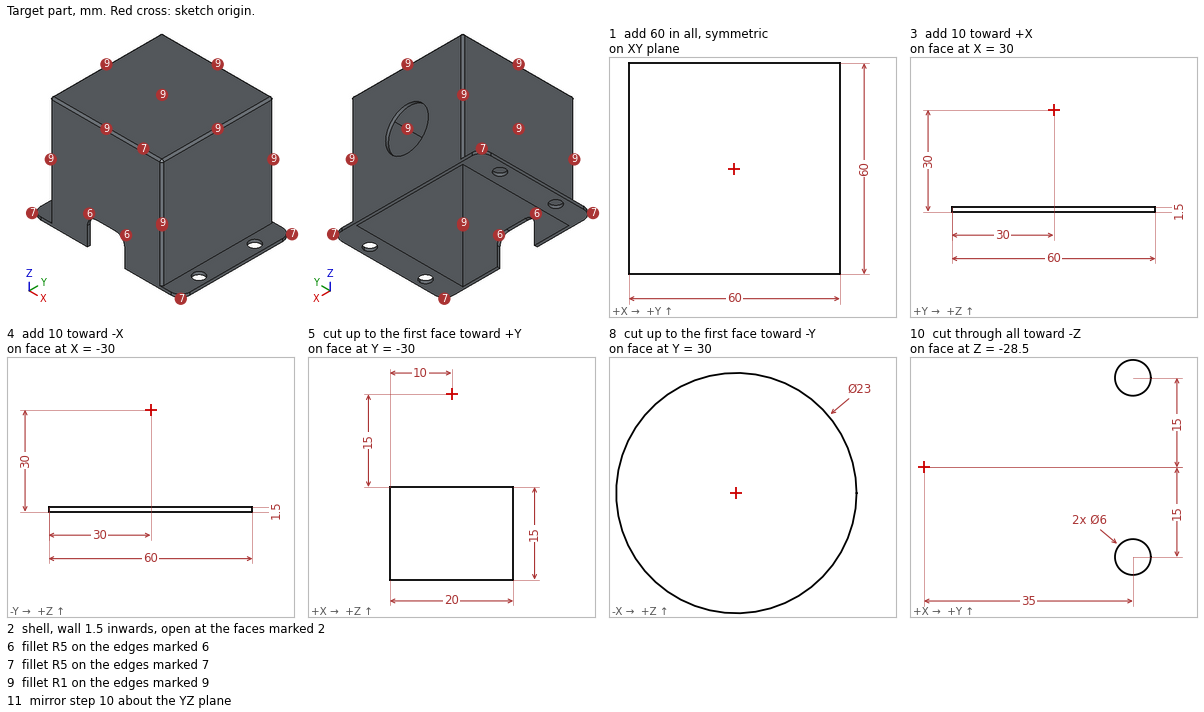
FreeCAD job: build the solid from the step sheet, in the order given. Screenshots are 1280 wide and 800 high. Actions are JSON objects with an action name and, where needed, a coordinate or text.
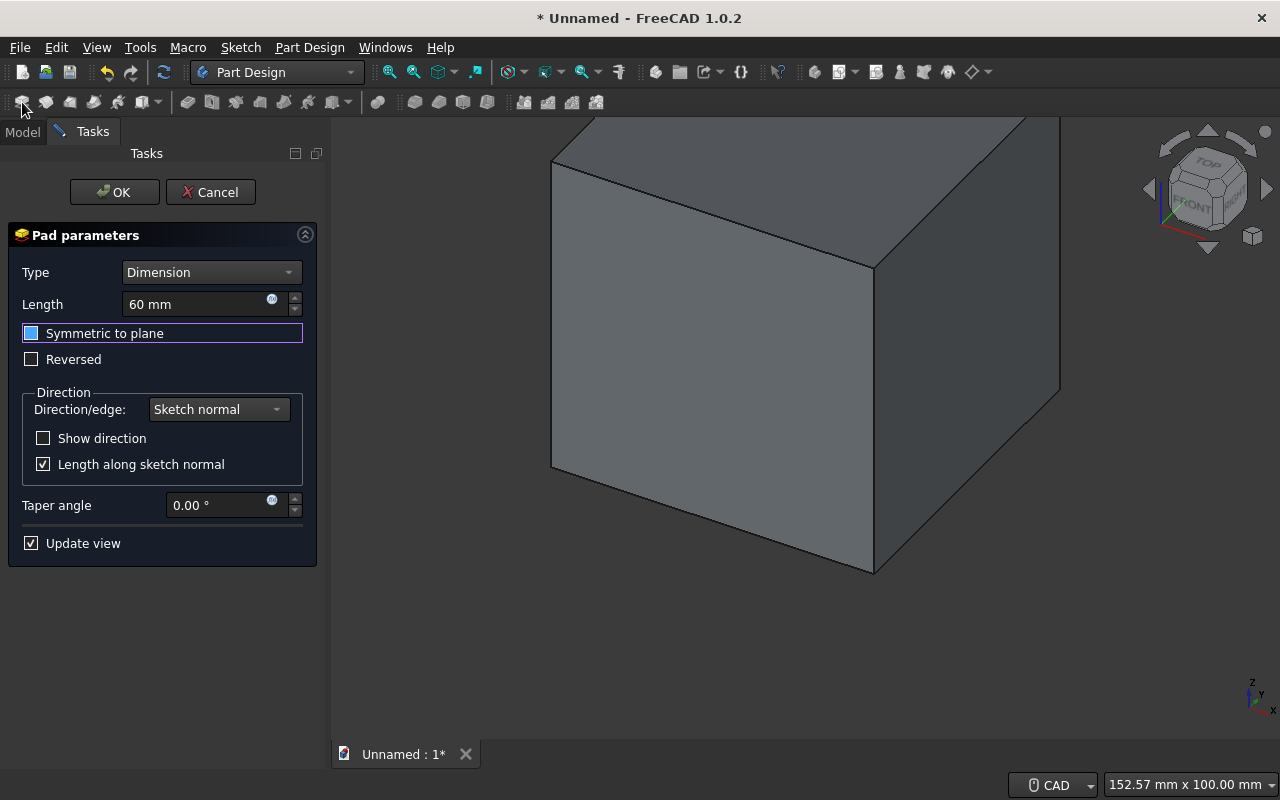
{"action": "left_click", "coordinate": [30, 333]}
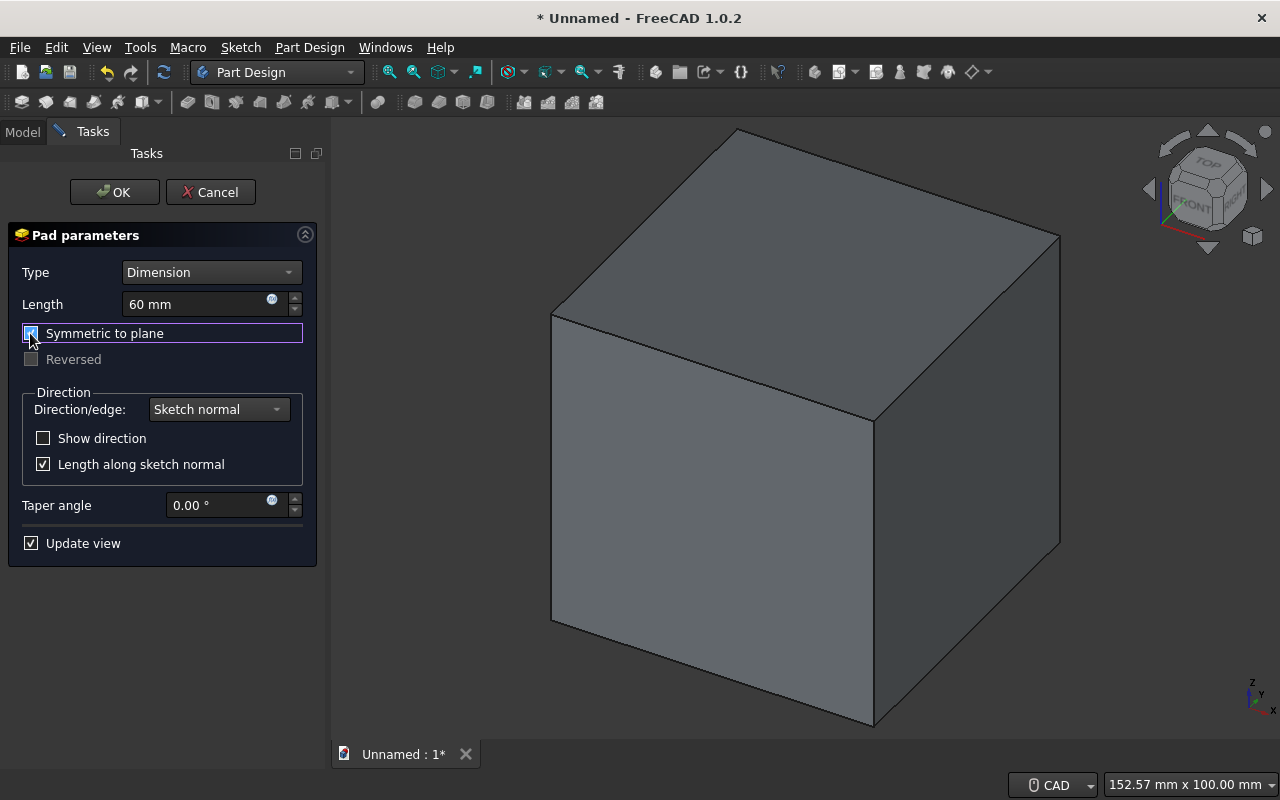
{"action": "left_click", "coordinate": [115, 192]}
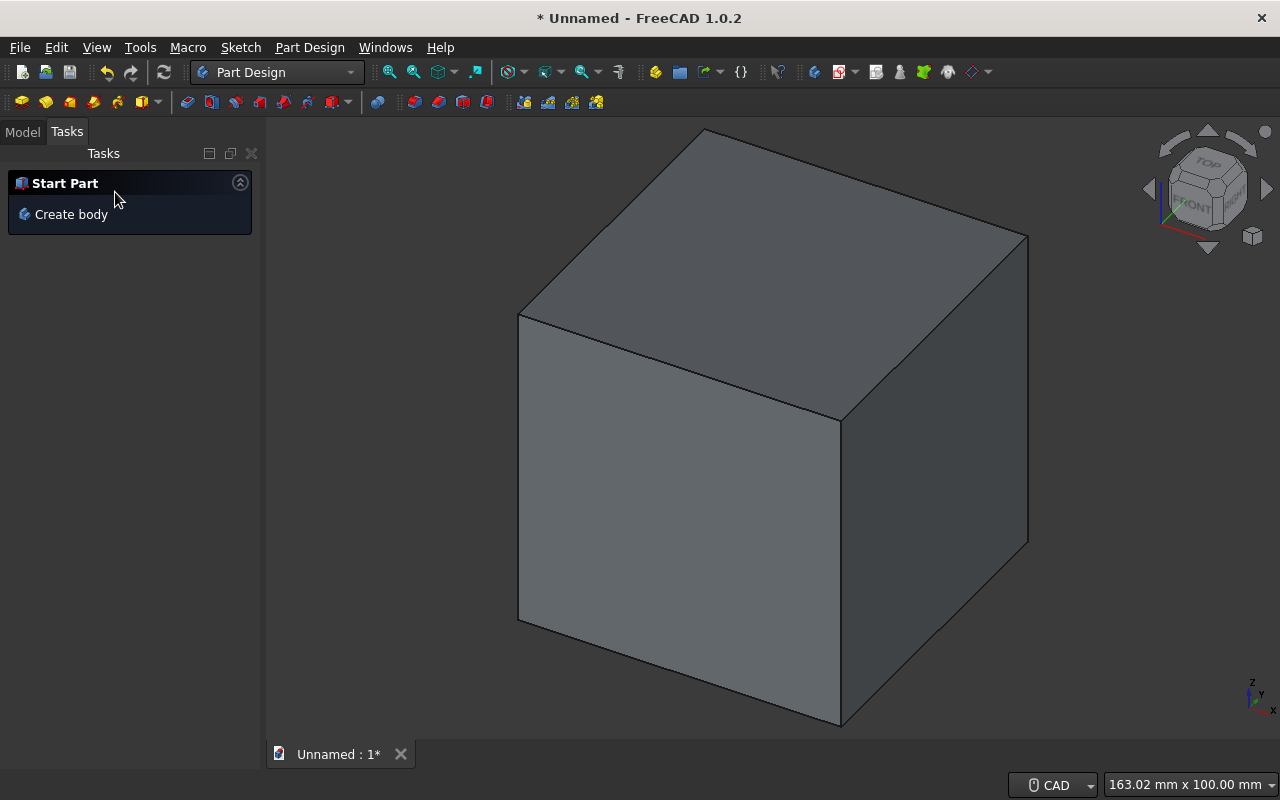
{"action": "key", "text": "0"}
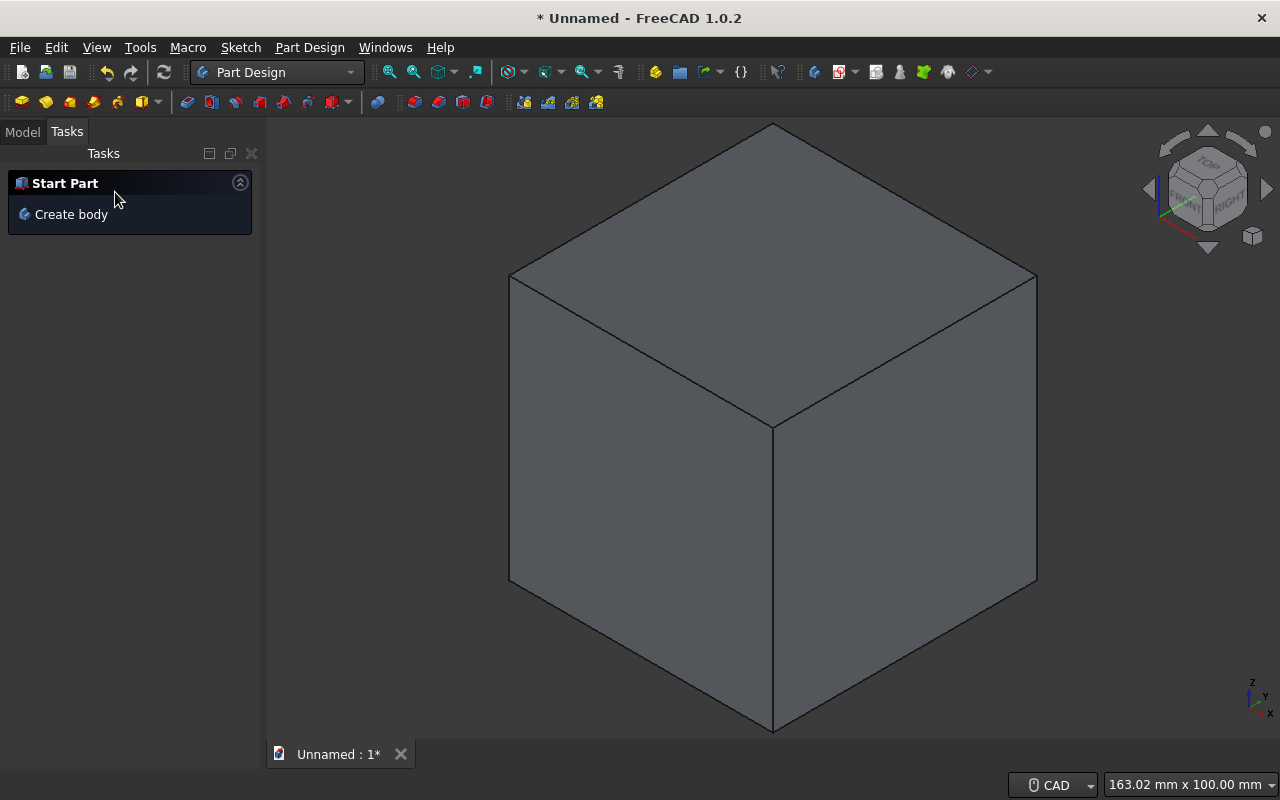
{"action": "key", "text": "2"}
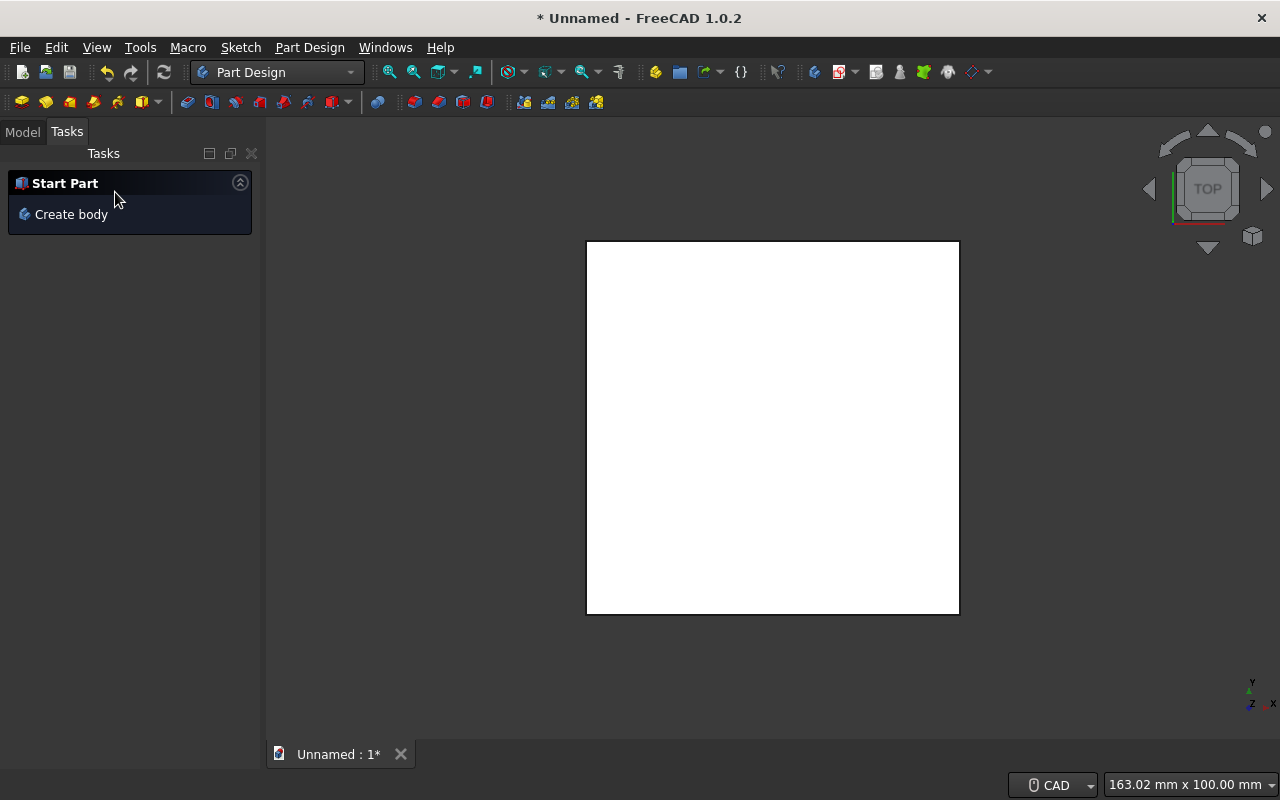
{"action": "key", "text": "1"}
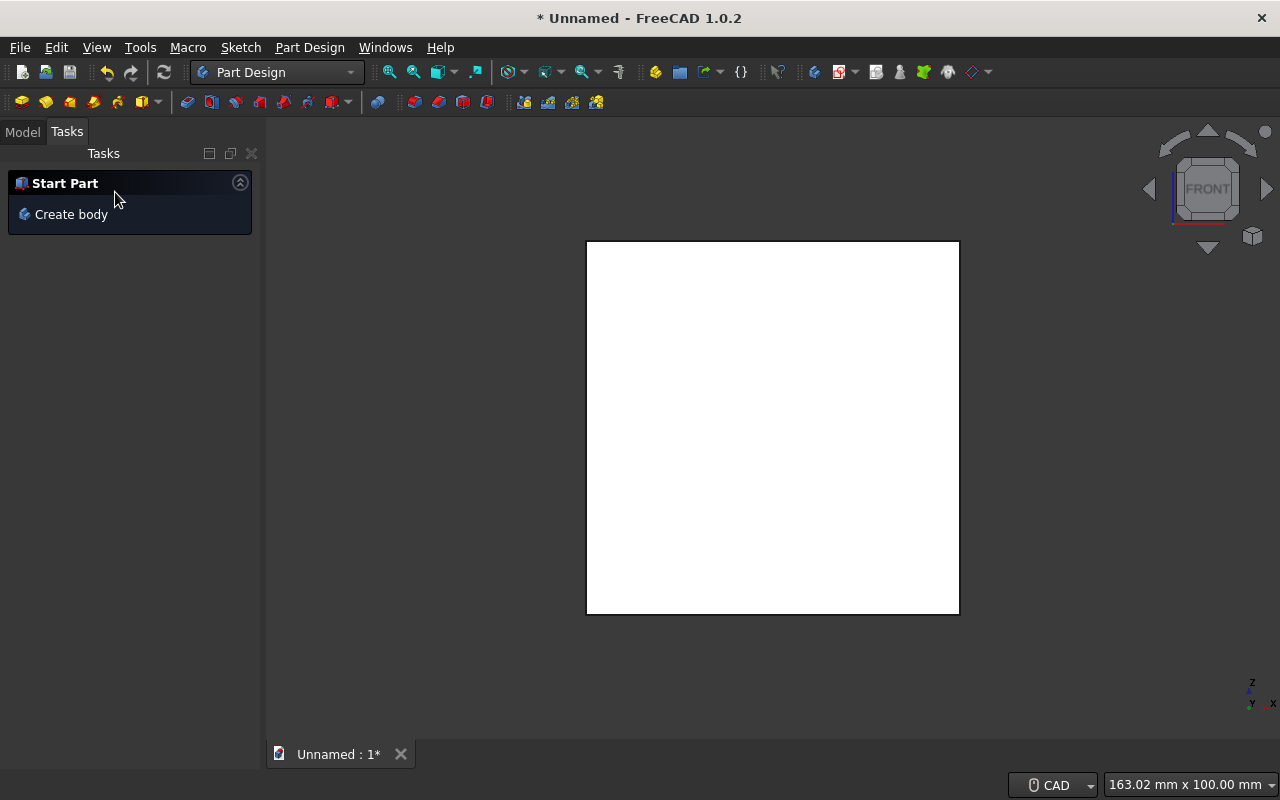
{"action": "key", "text": "3"}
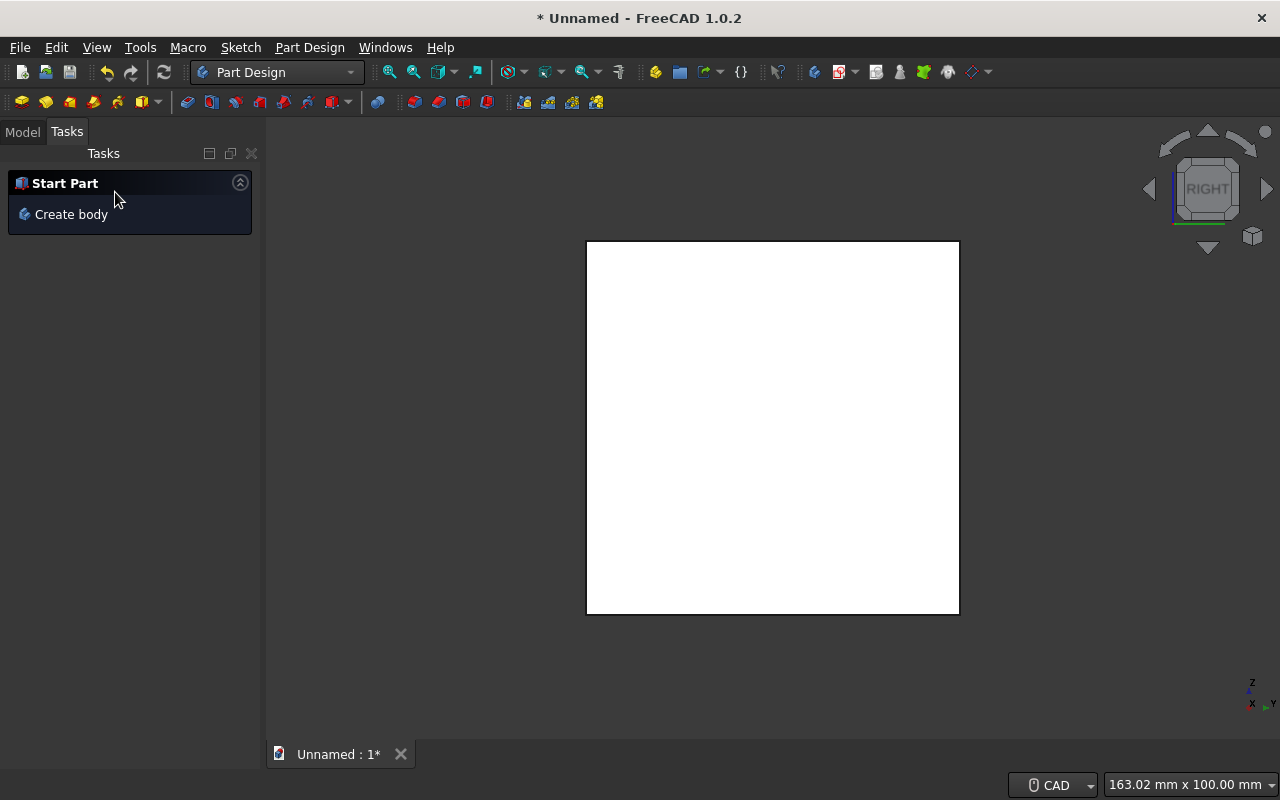
{"action": "key", "text": "5"}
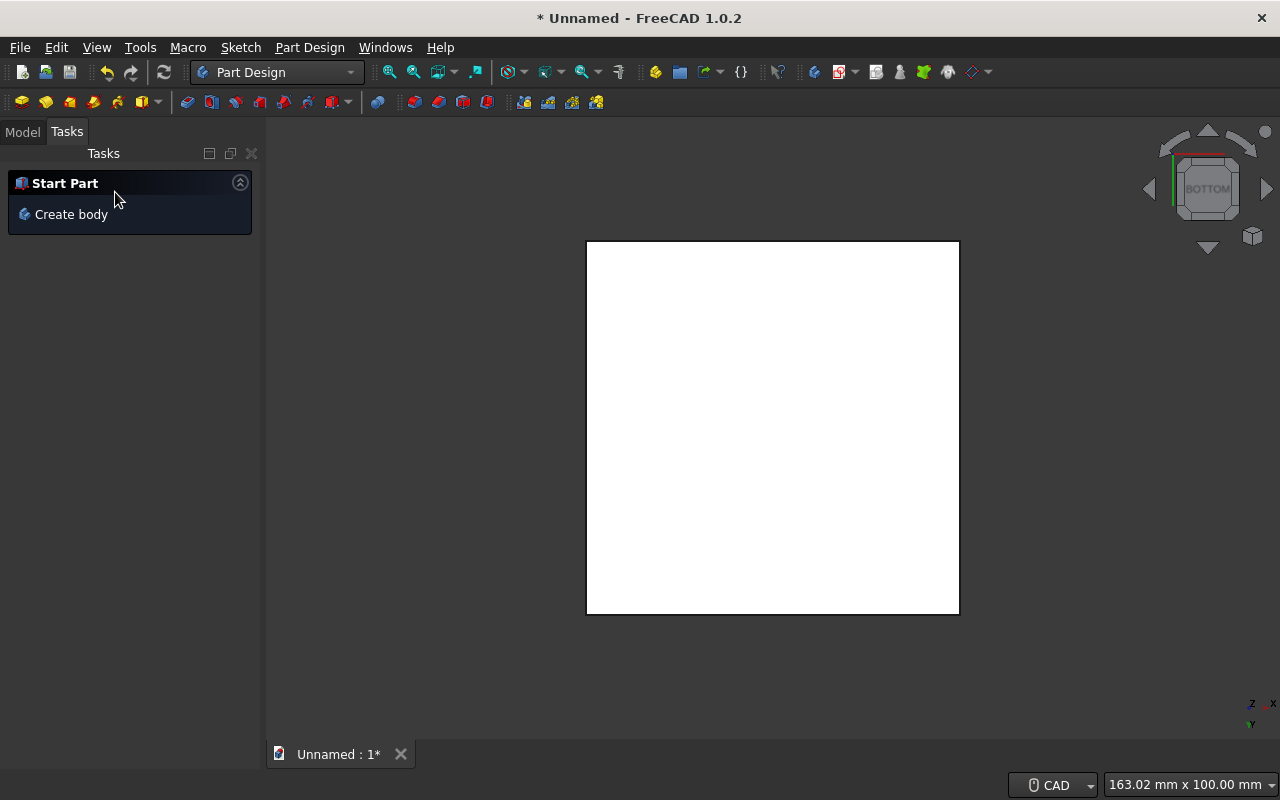
{"action": "left_click", "coordinate": [773, 427]}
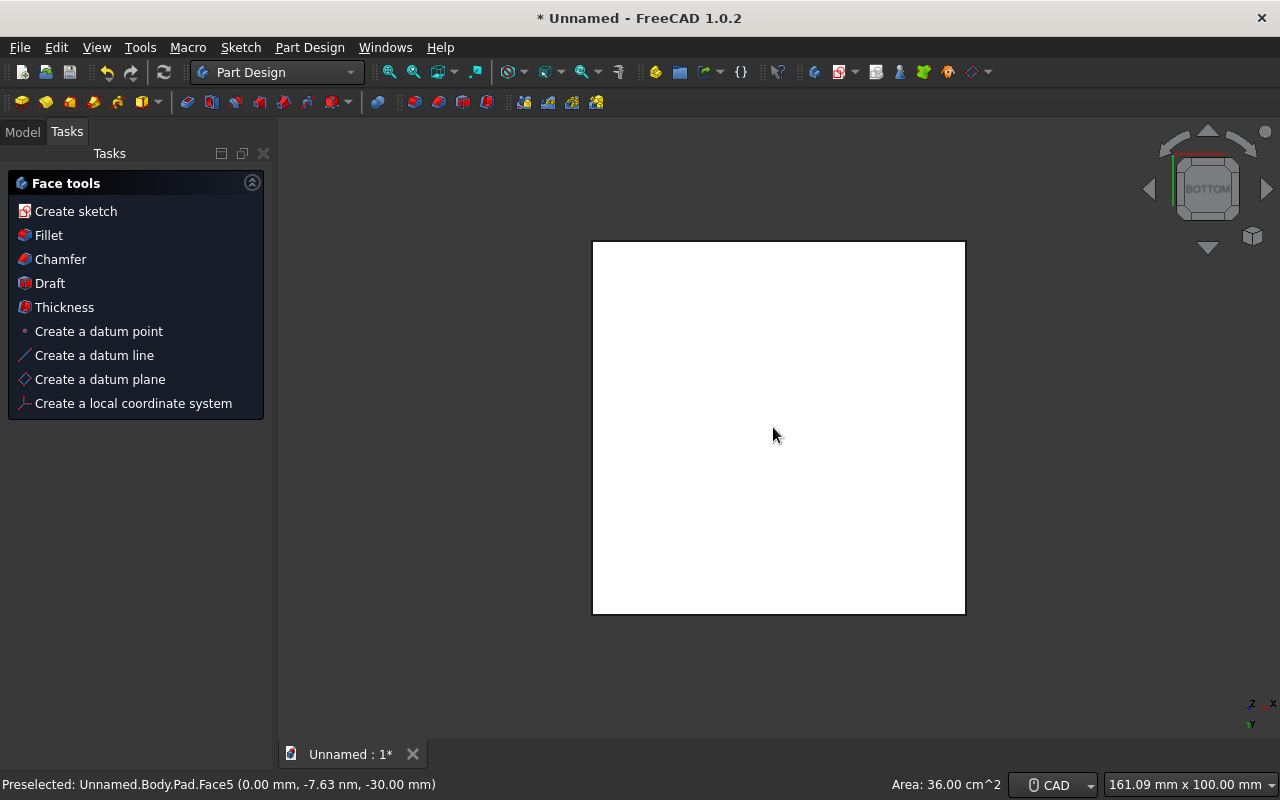
{"action": "left_click", "coordinate": [488, 102]}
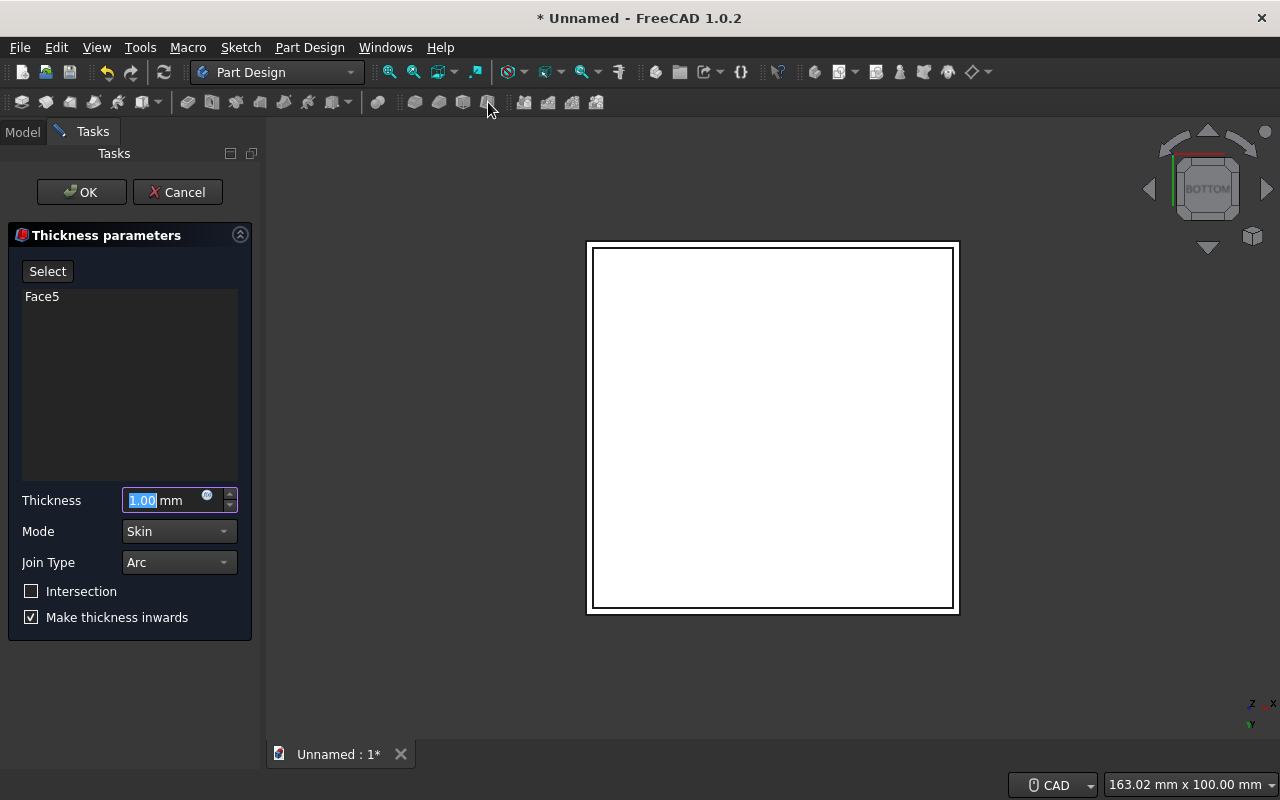
{"action": "type", "text": "1.5"}
{"action": "key", "text": "Tab"}